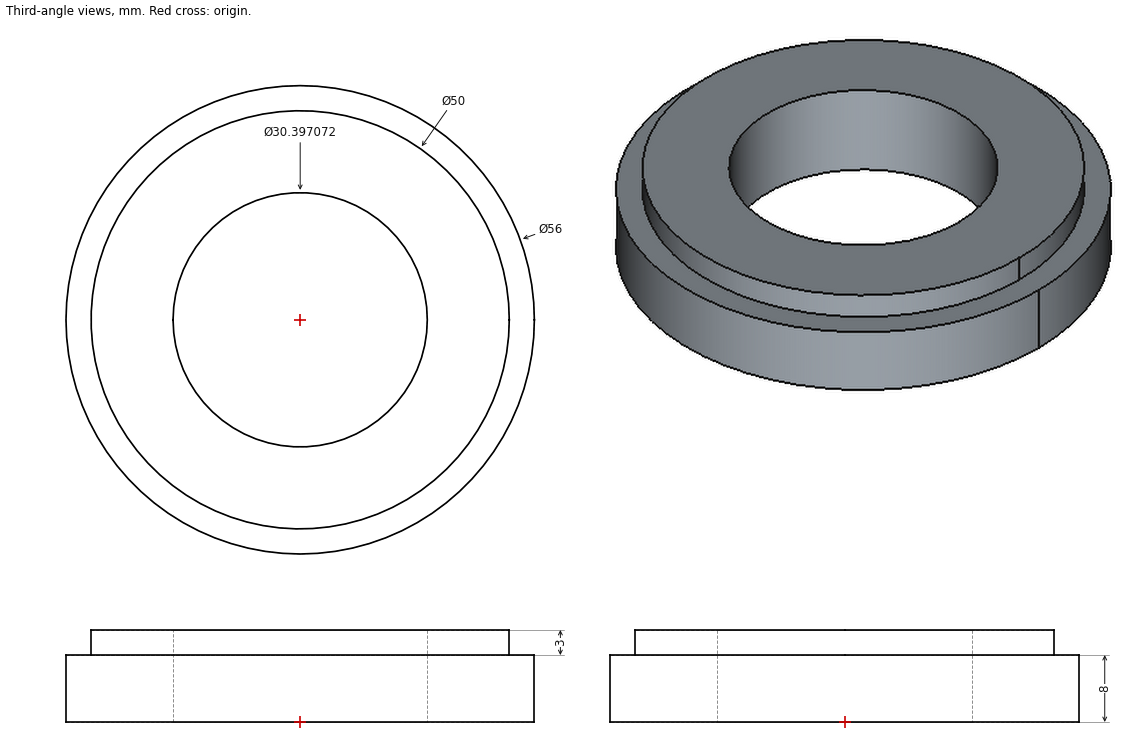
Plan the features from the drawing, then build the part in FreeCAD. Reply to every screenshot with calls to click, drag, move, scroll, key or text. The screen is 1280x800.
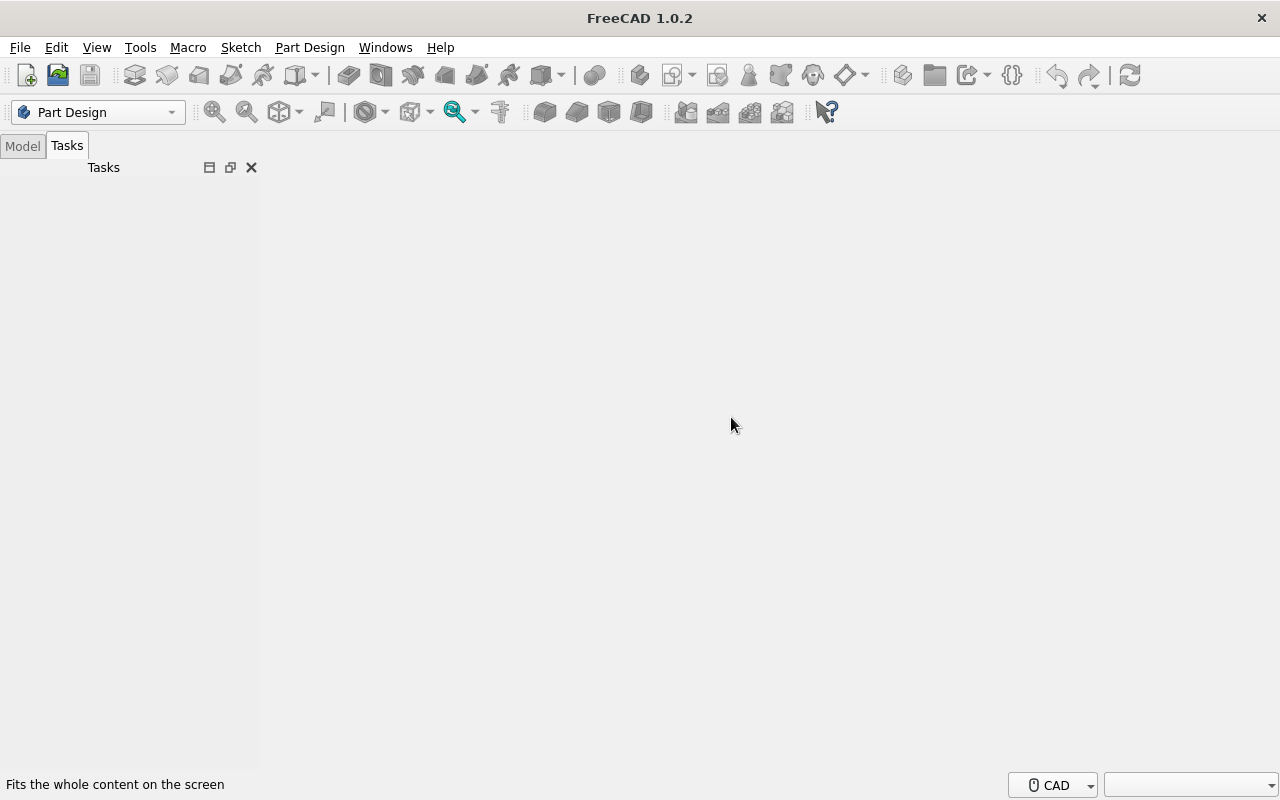
click(26, 76)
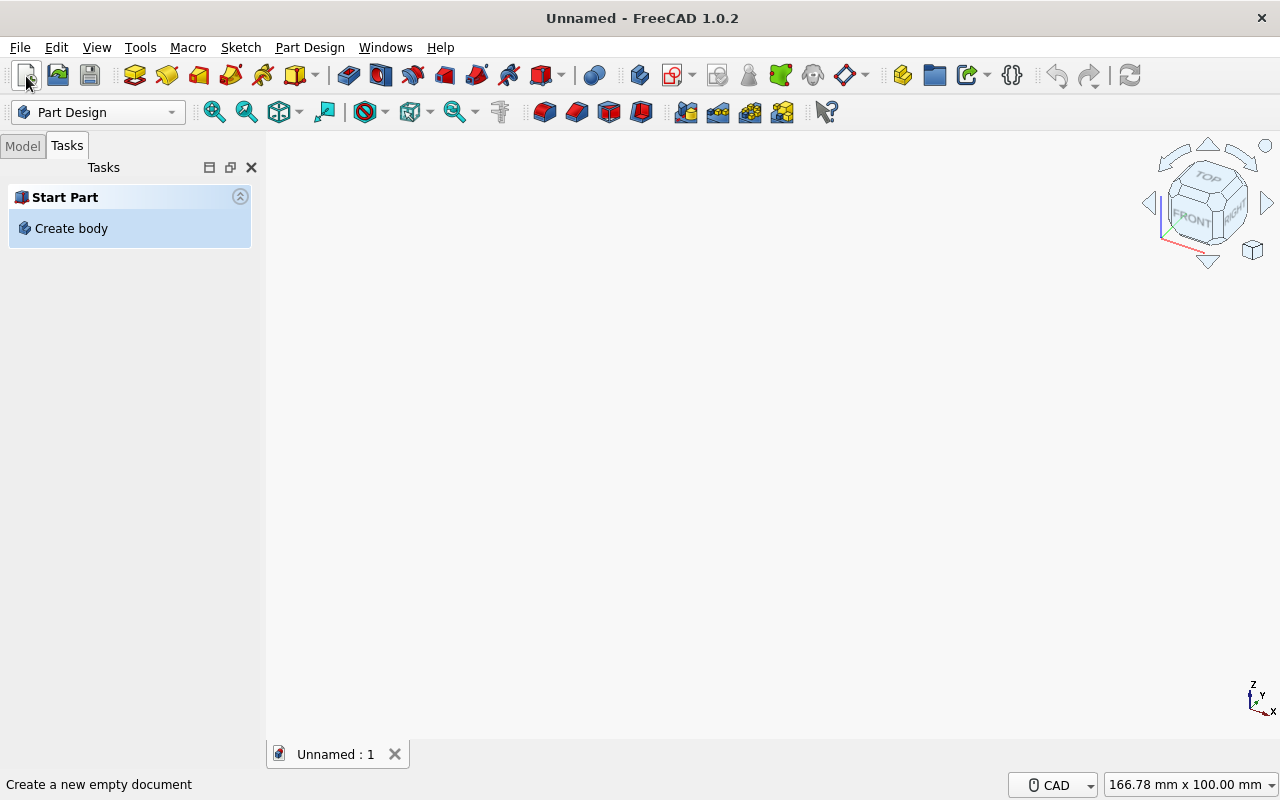
click(672, 76)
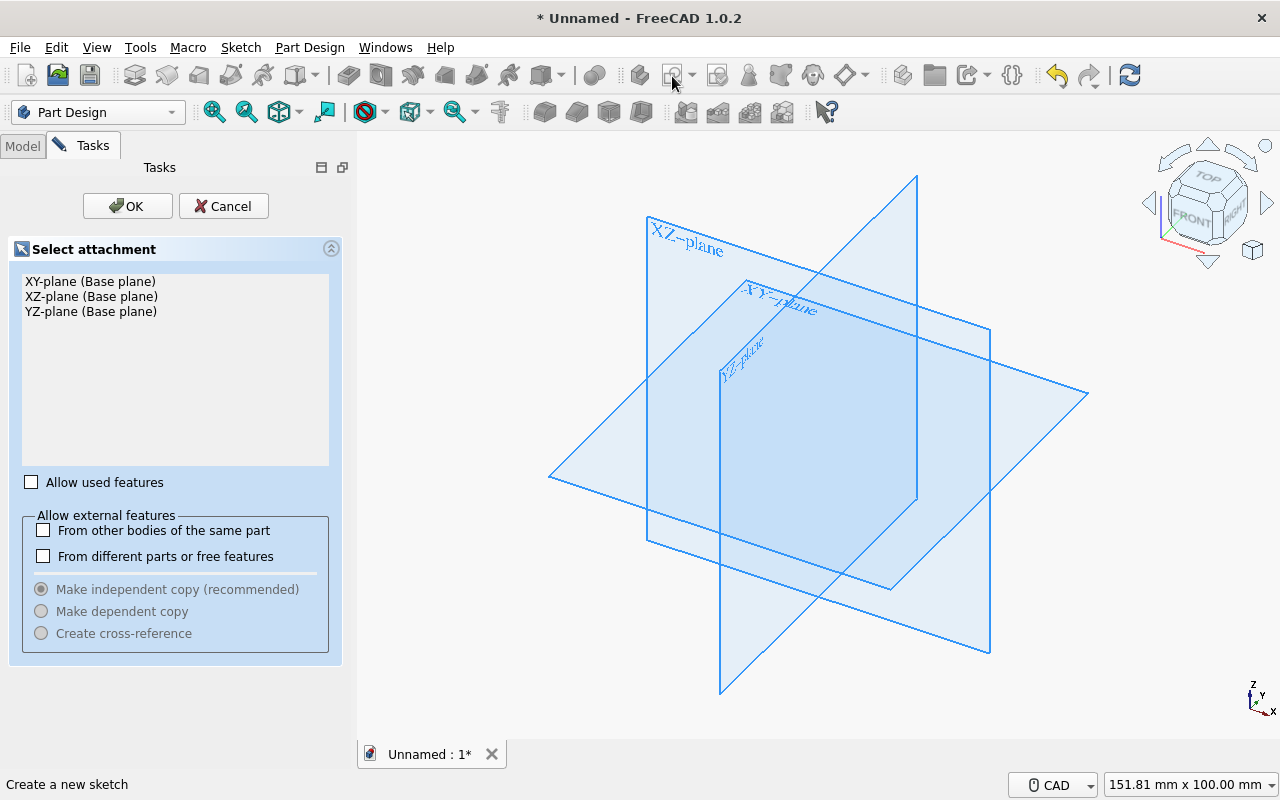
click(82, 282)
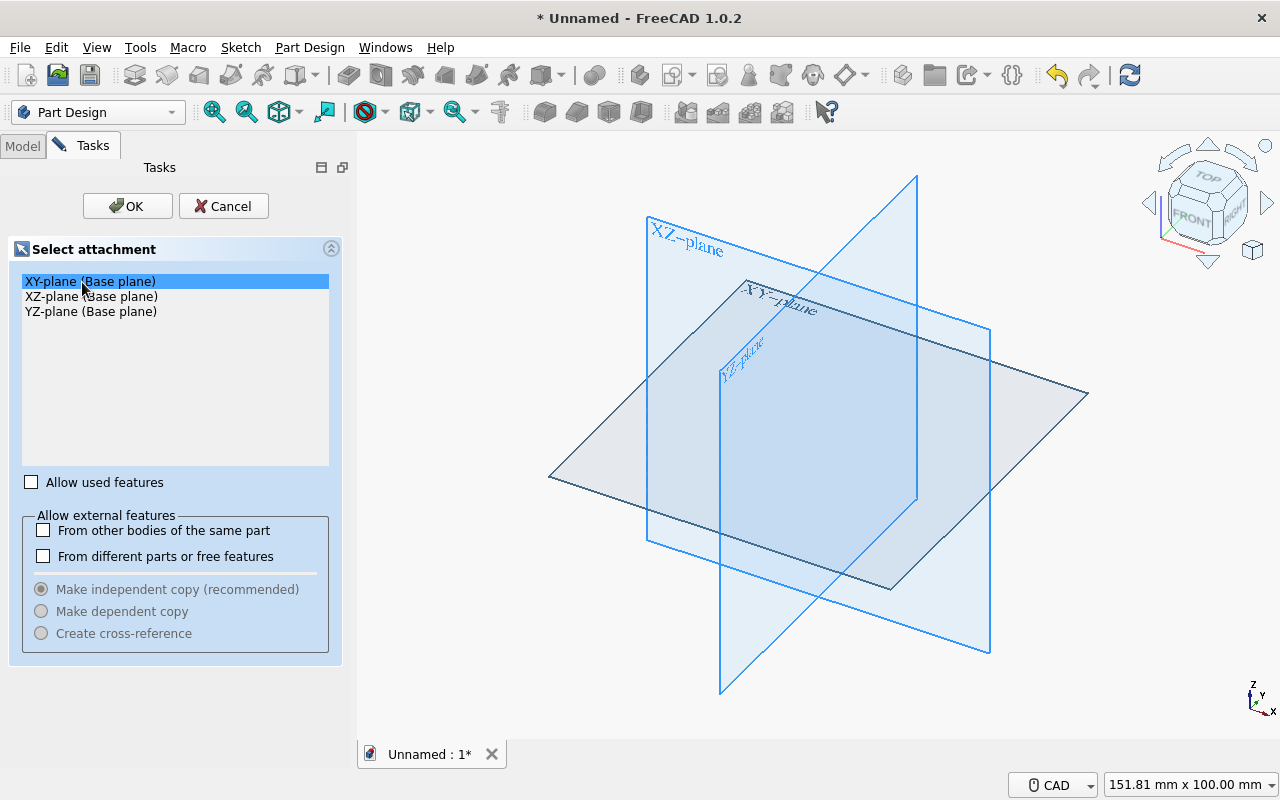
click(128, 206)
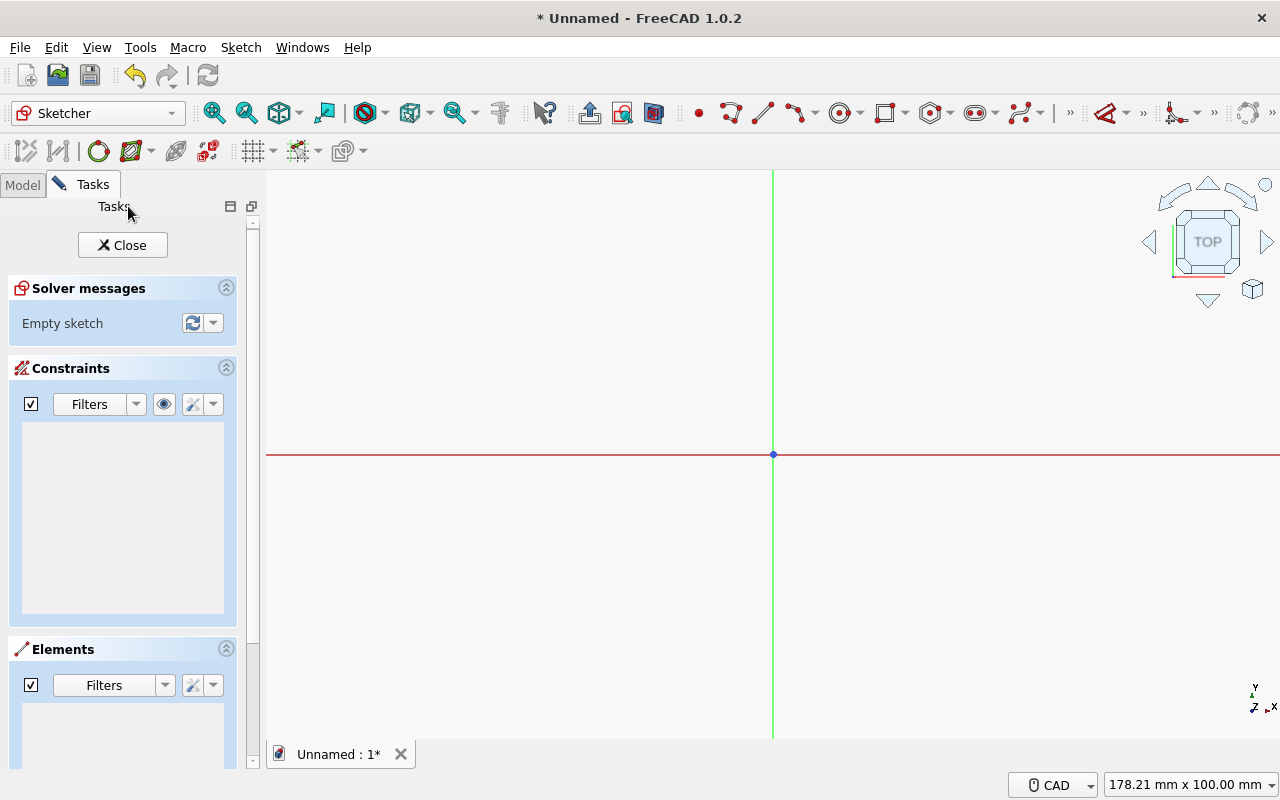
key(g)
key(c)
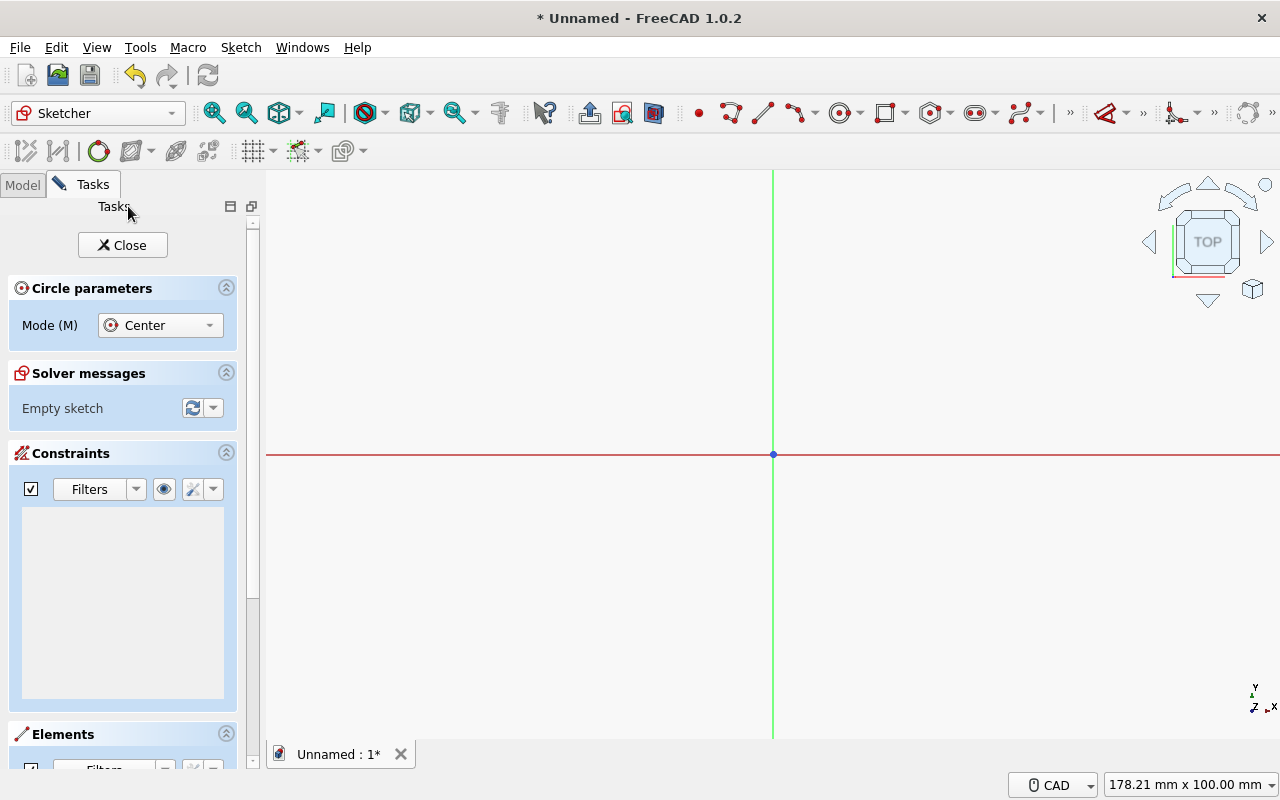
click(773, 454)
click(886, 342)
key(Escape)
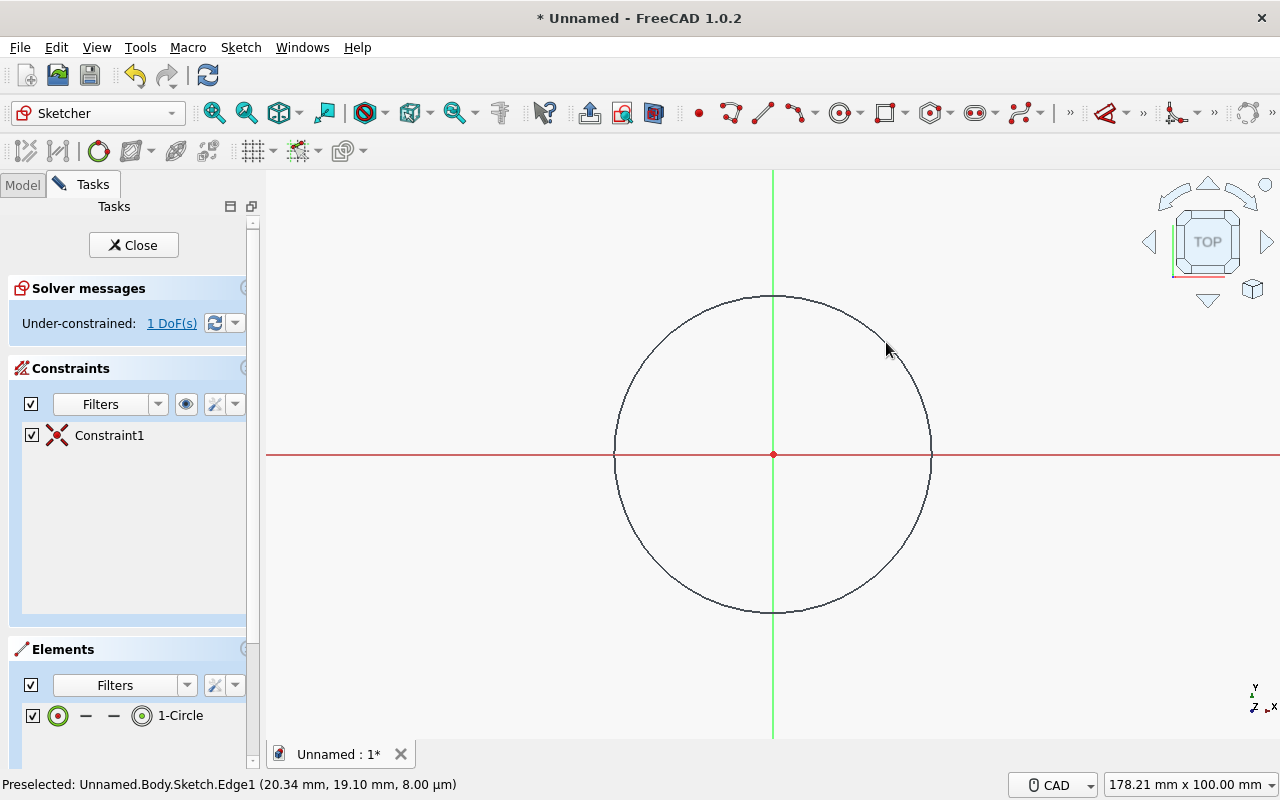
click(1106, 114)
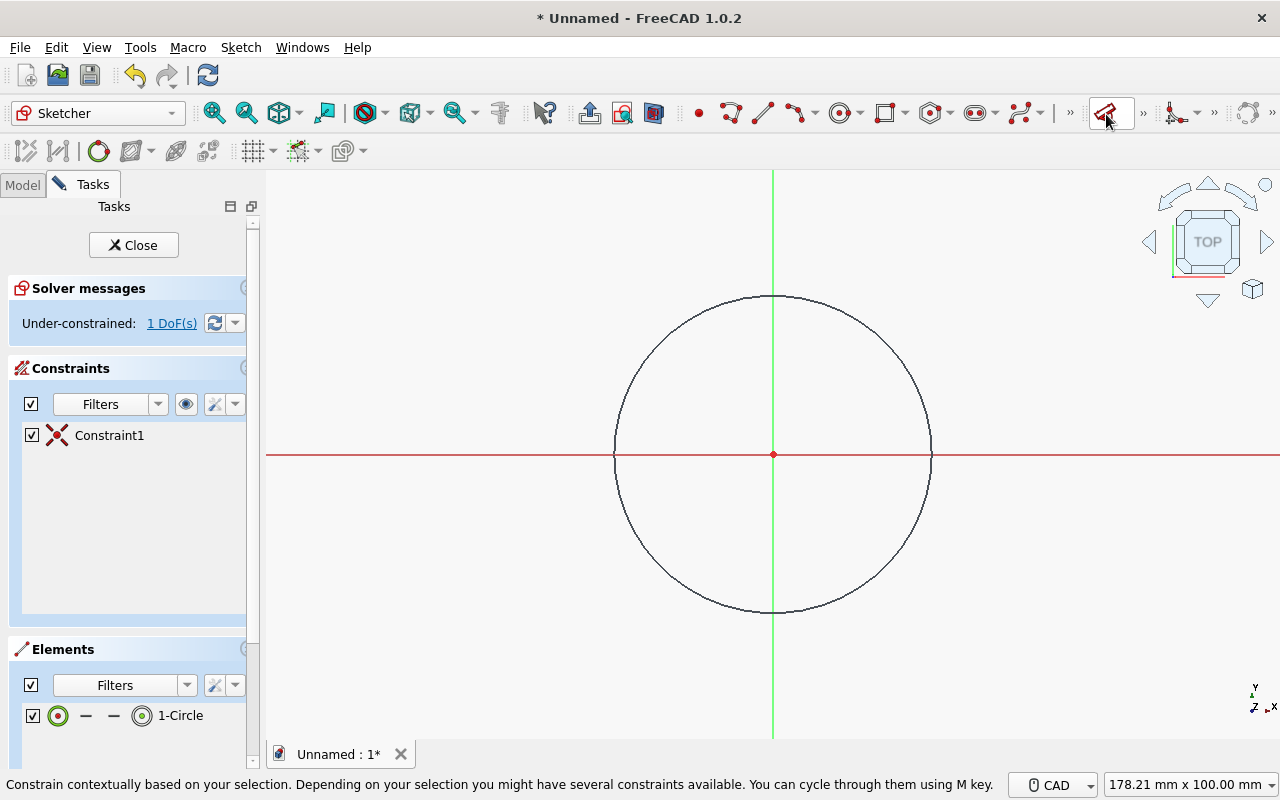
click(885, 342)
click(908, 319)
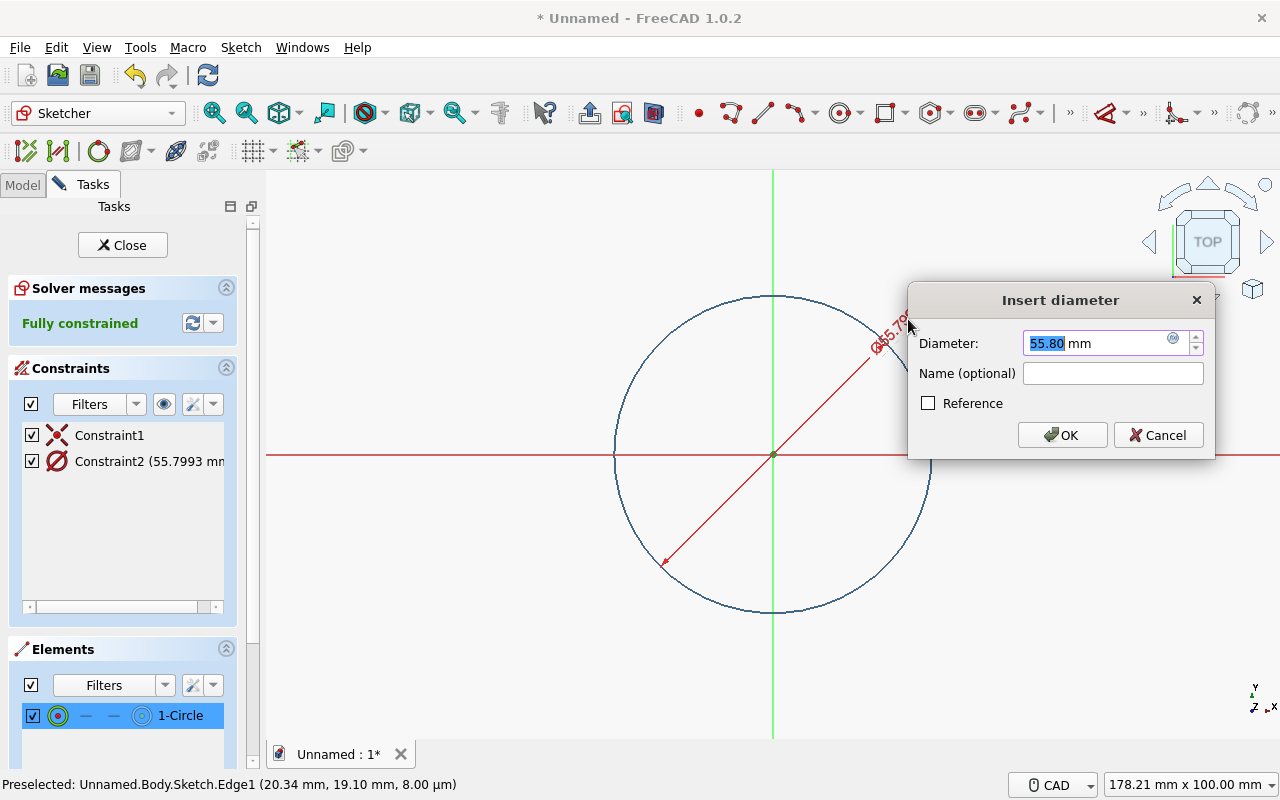
text(56)
key(Return)
key(Escape)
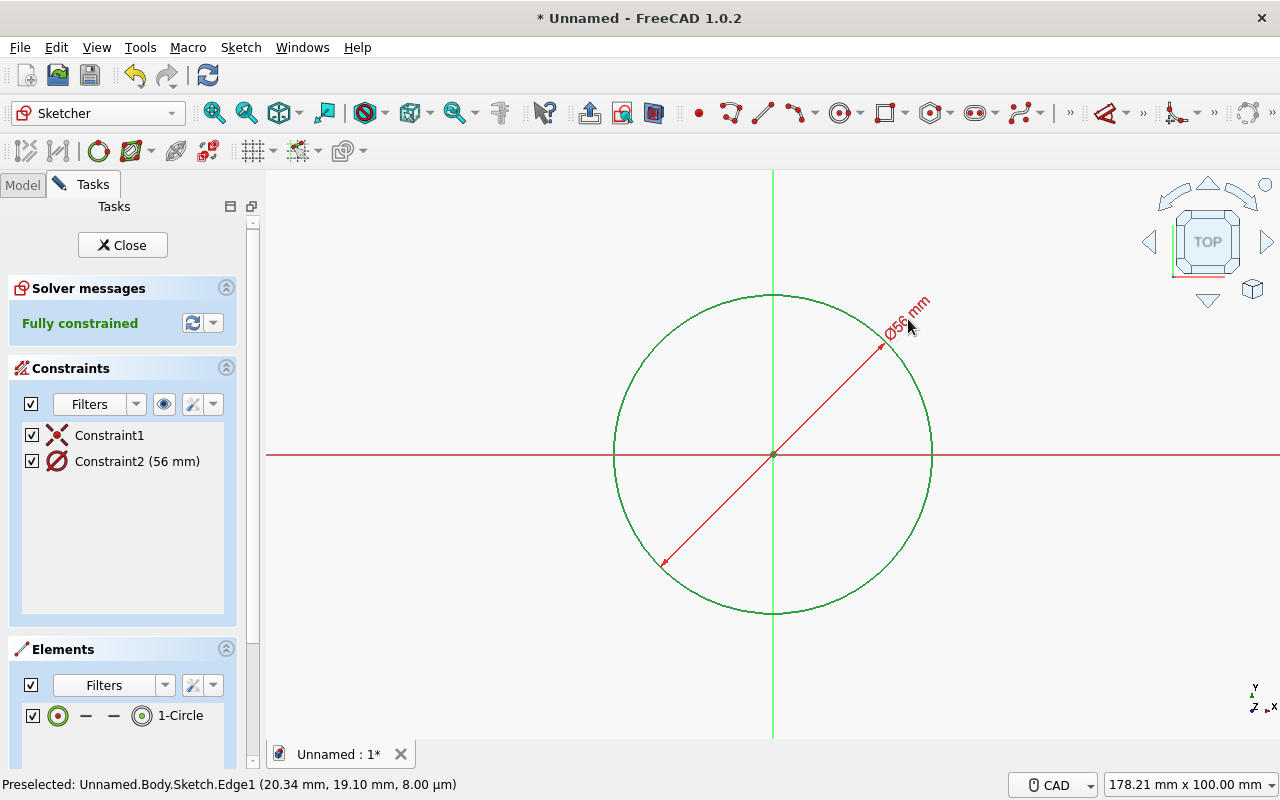
click(123, 245)